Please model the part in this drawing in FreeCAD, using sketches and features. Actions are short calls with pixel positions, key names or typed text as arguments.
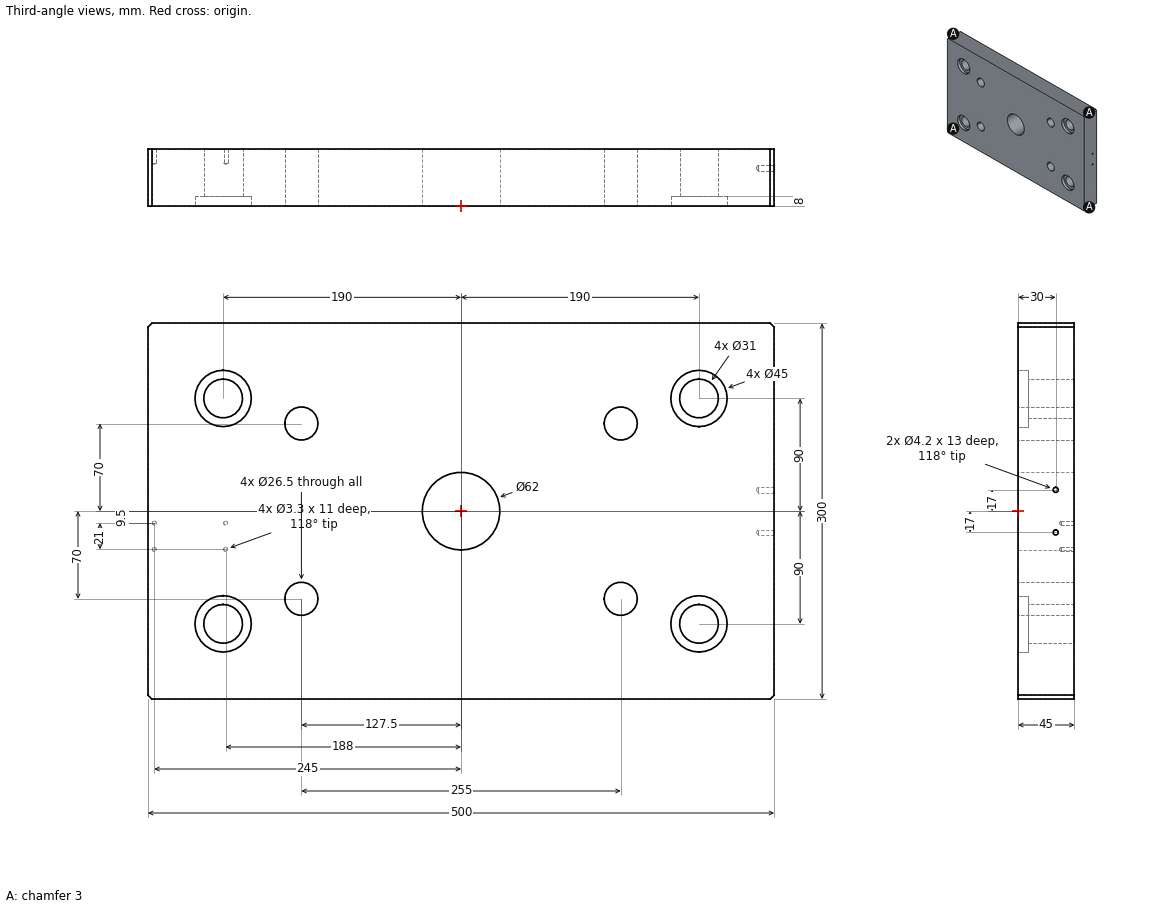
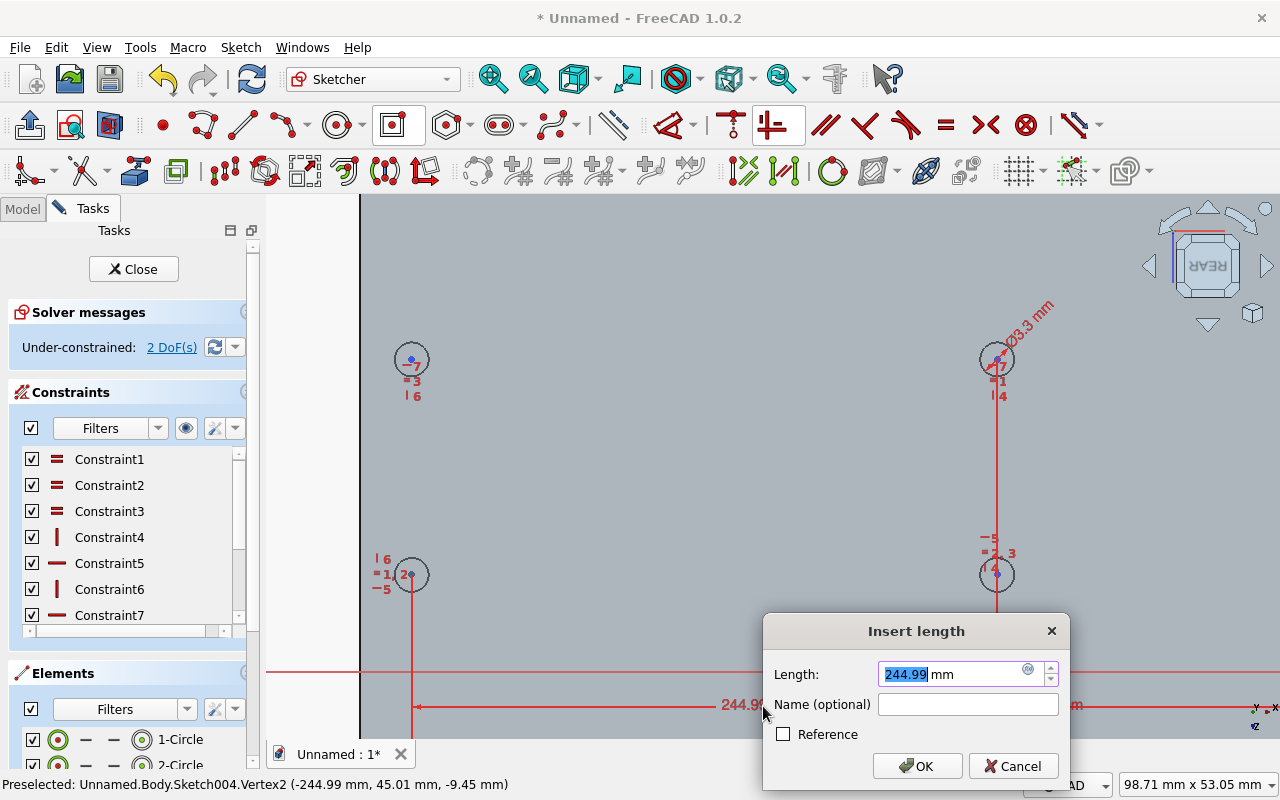
text(245)
key(Return)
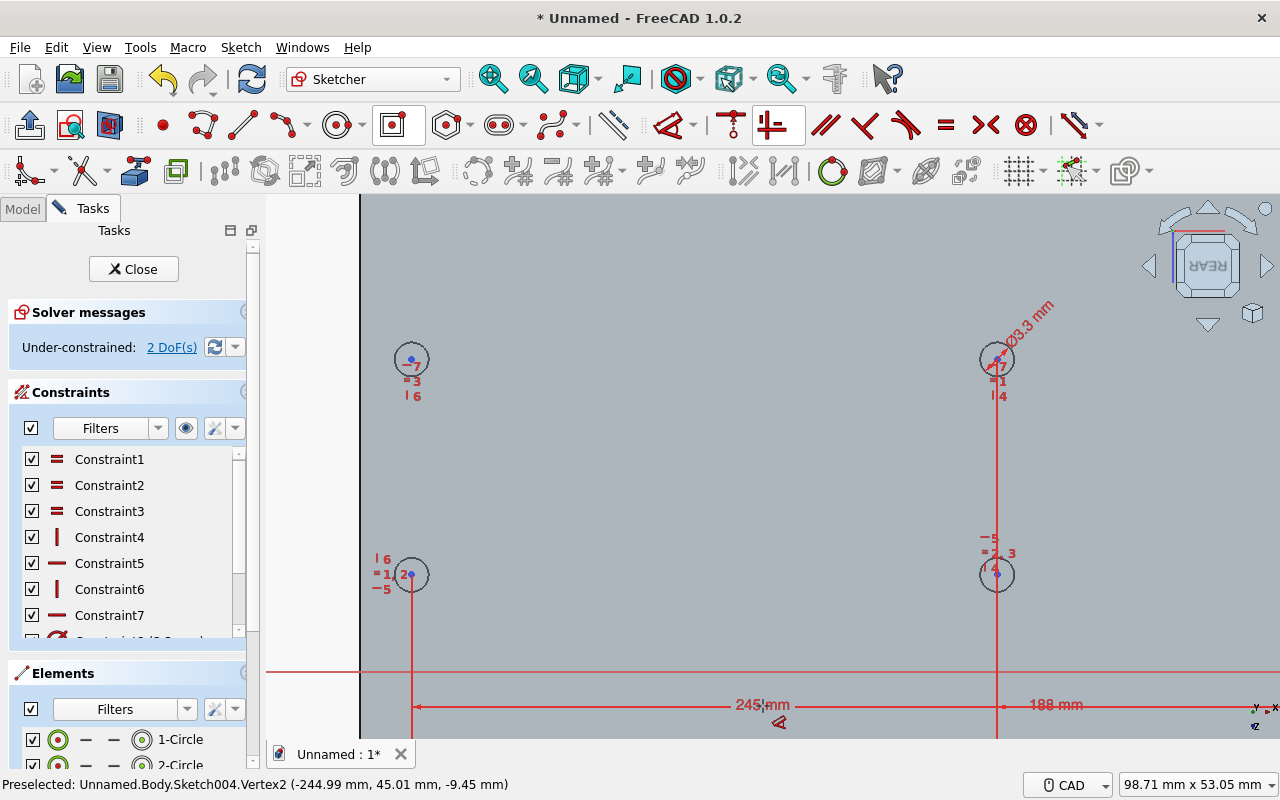
click(412, 575)
click(378, 623)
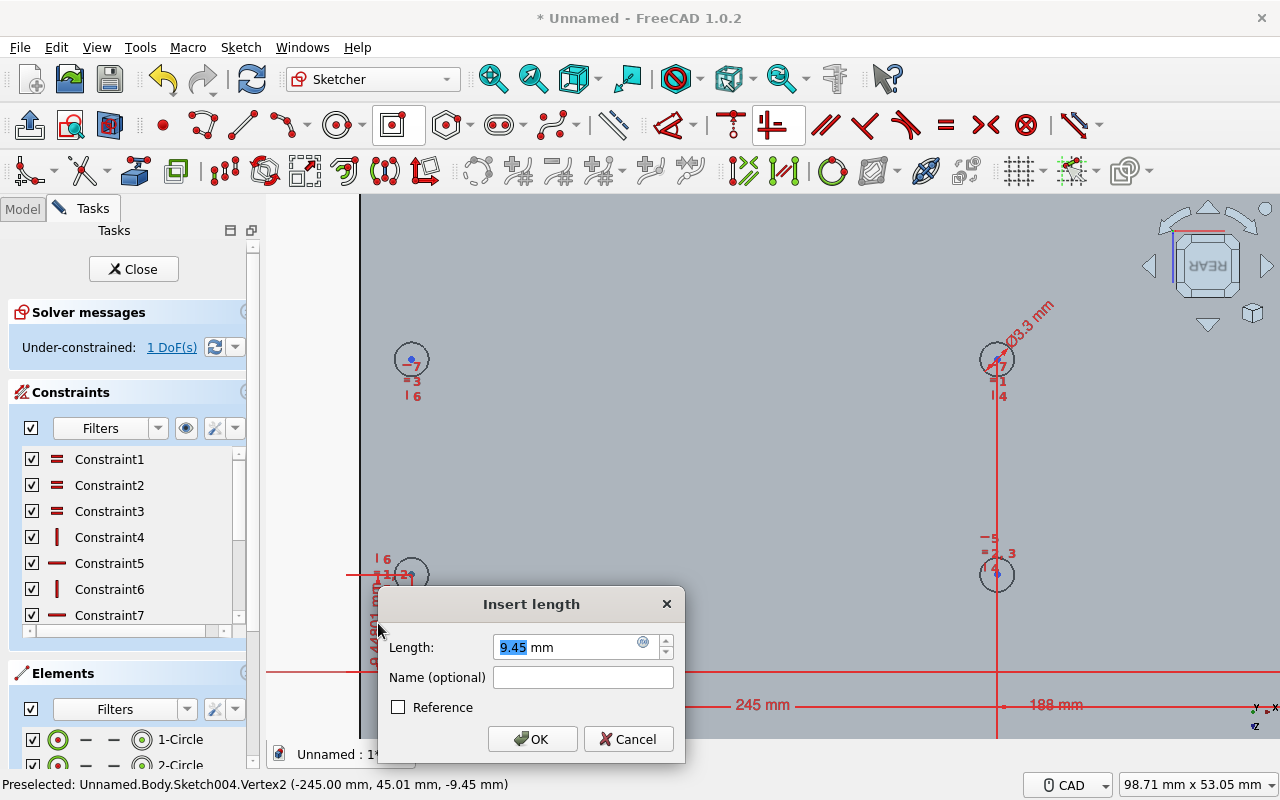
text(9.5)
key(Return)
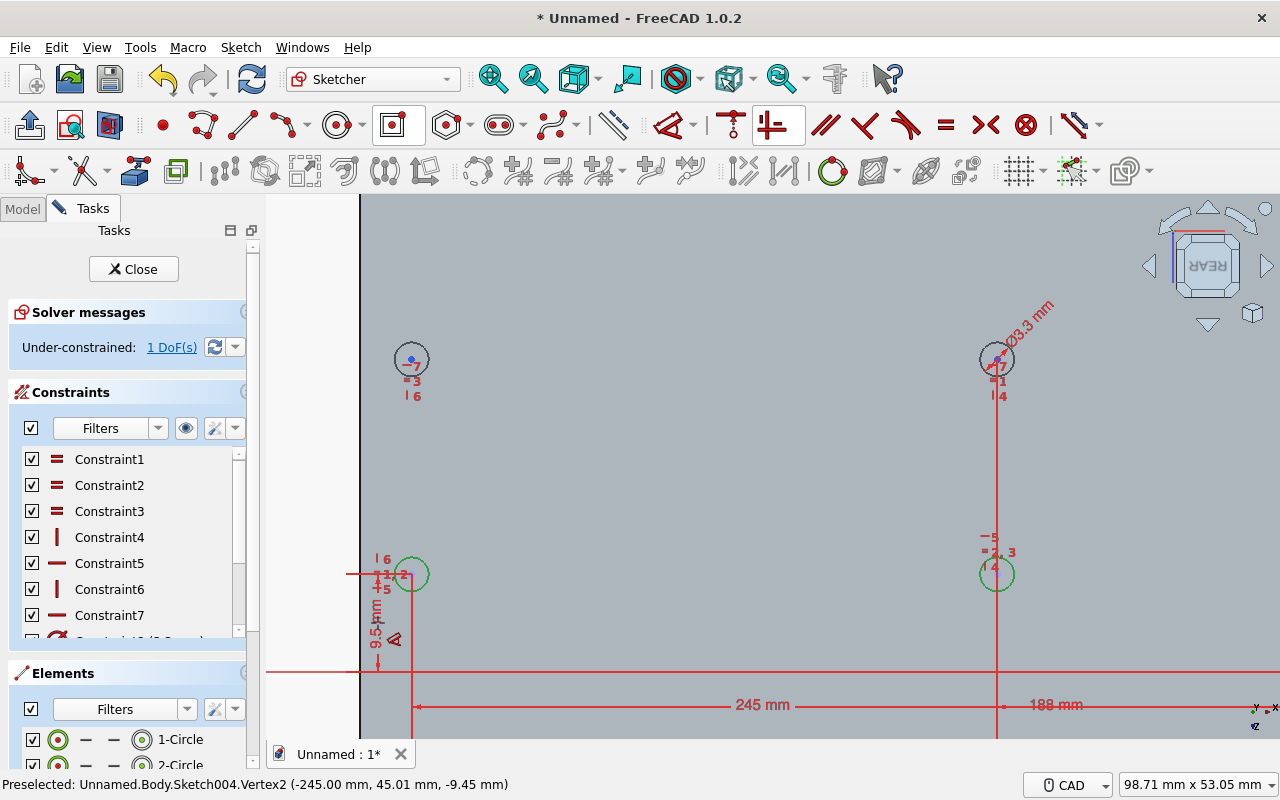
click(997, 359)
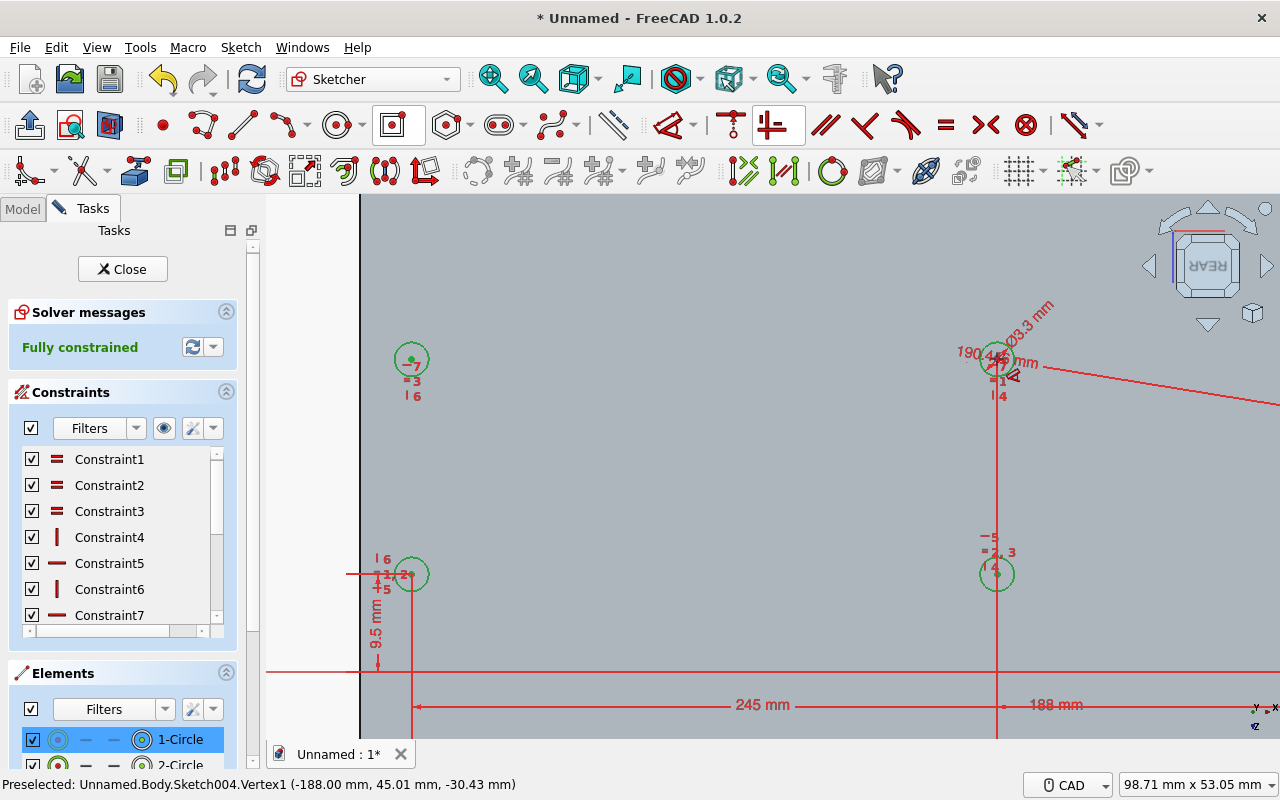
click(412, 574)
click(378, 467)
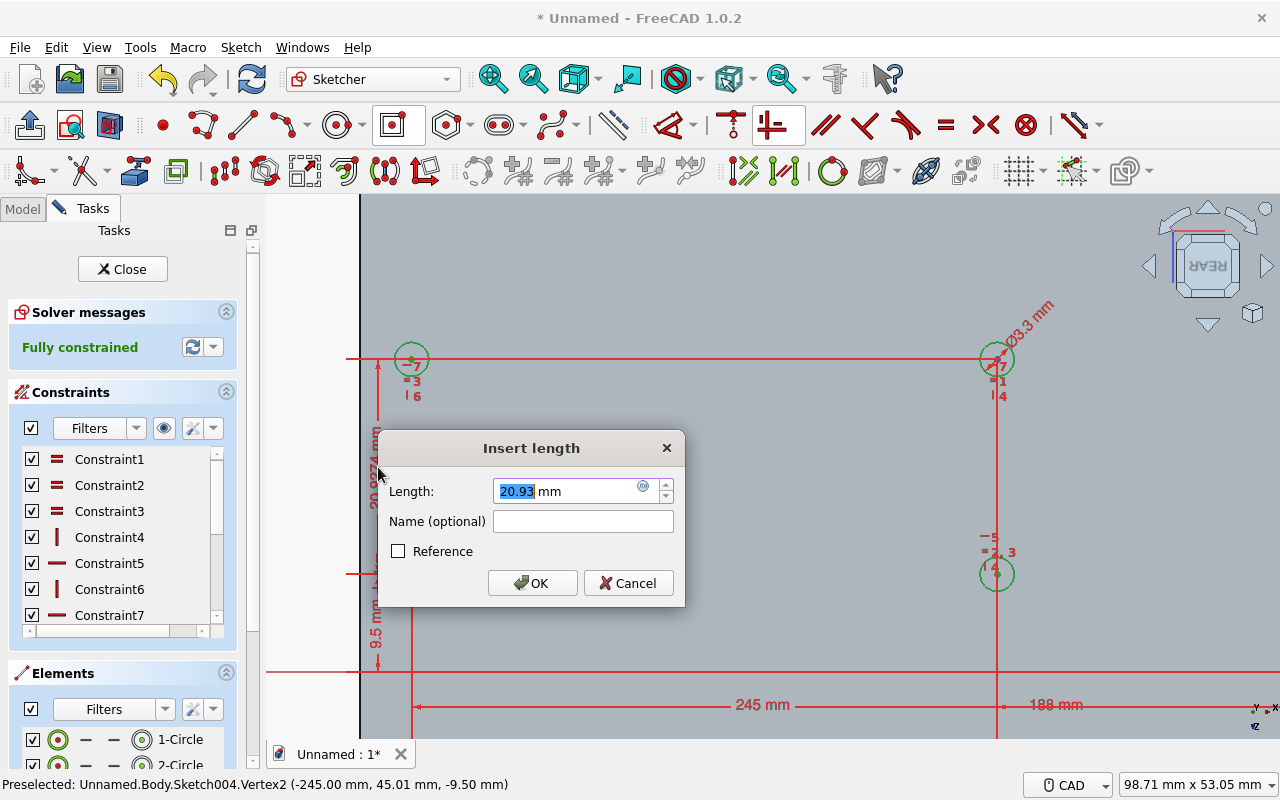
text(21)
key(Return)
key(Escape)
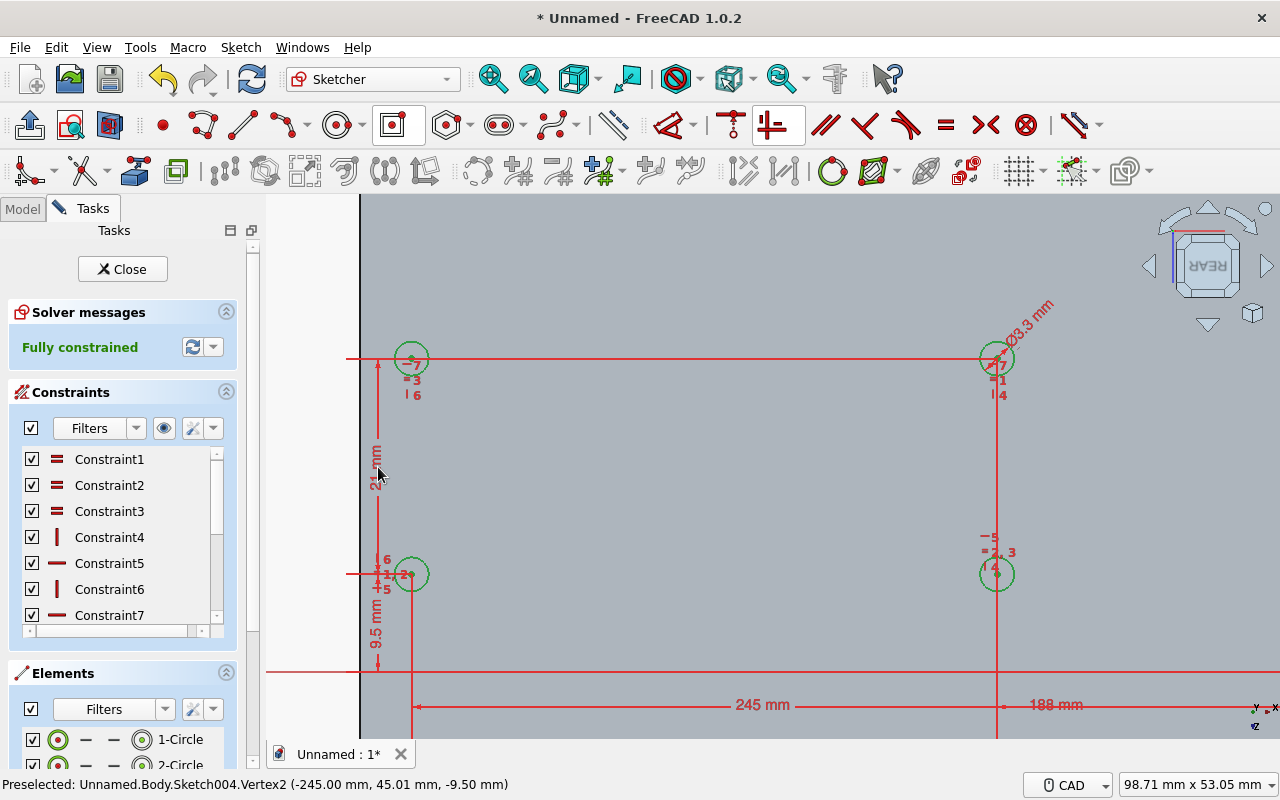
click(123, 269)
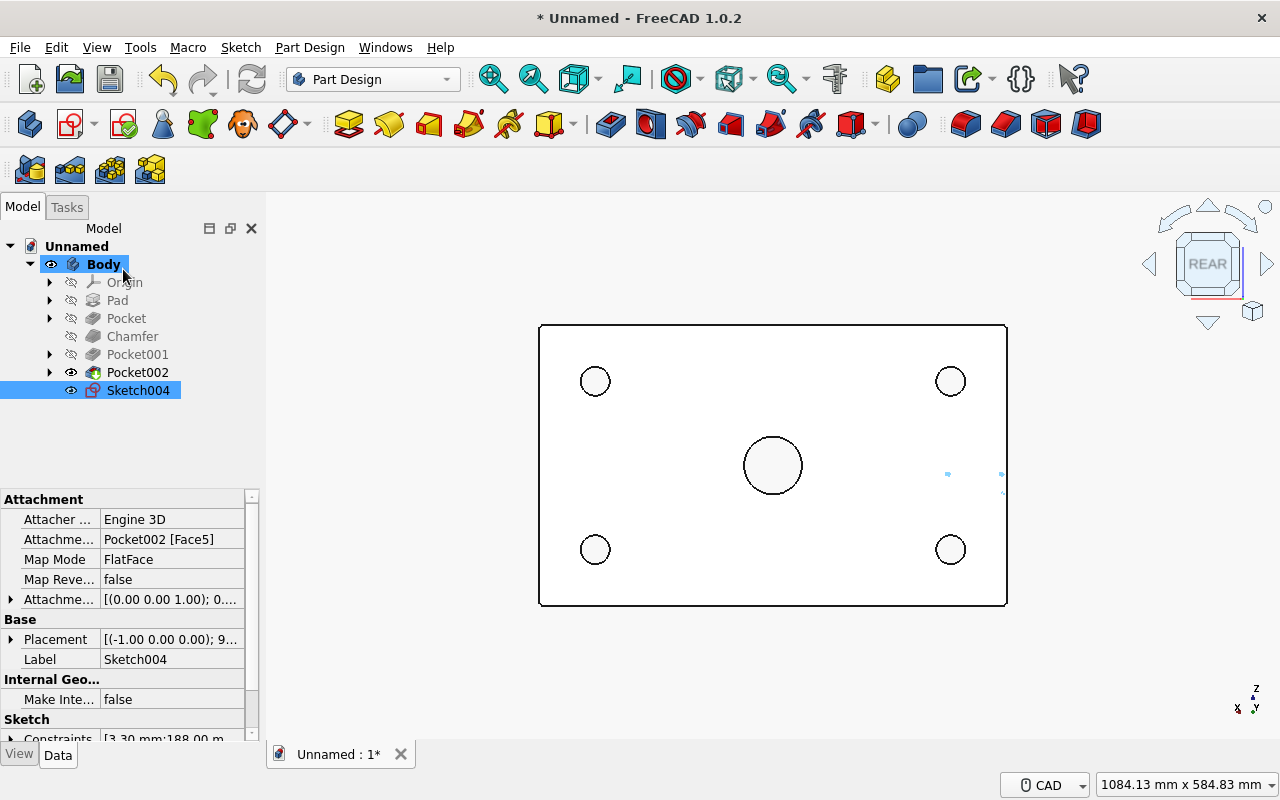
click(652, 124)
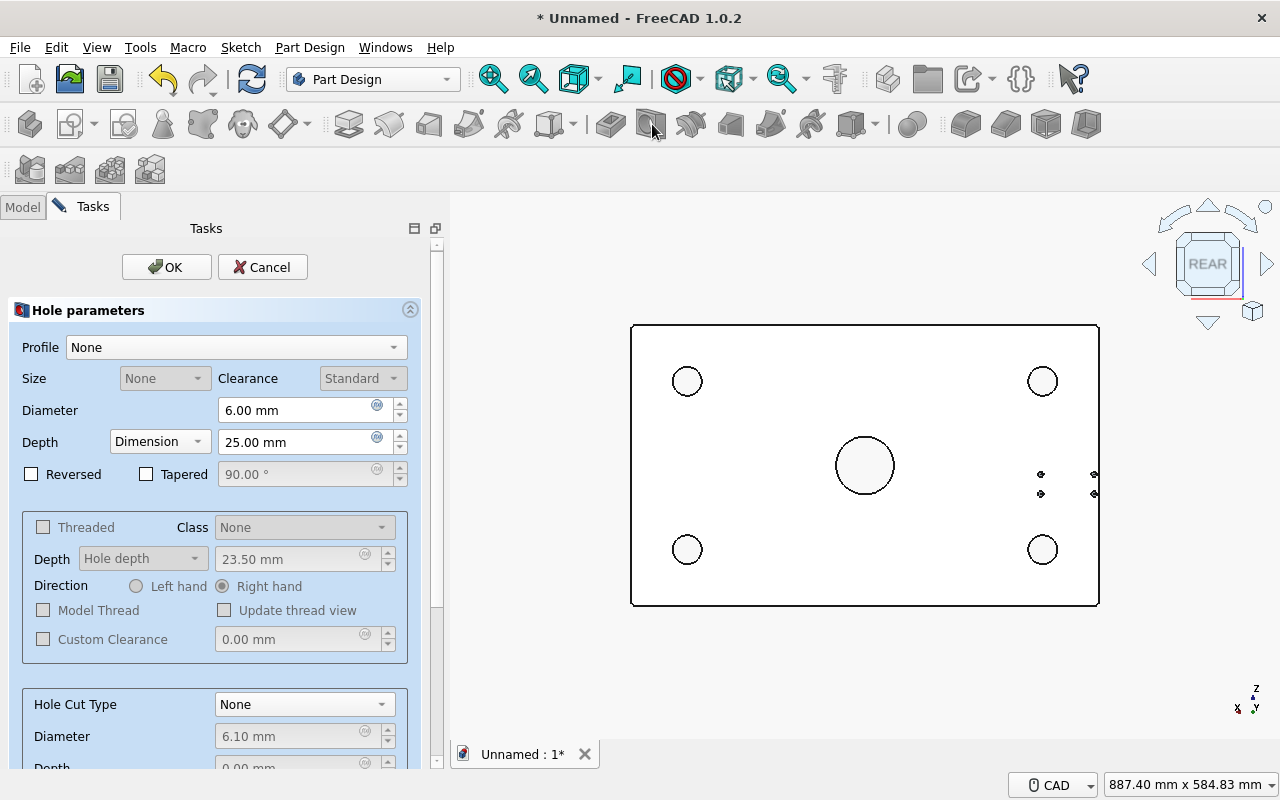
triple_click(305, 410)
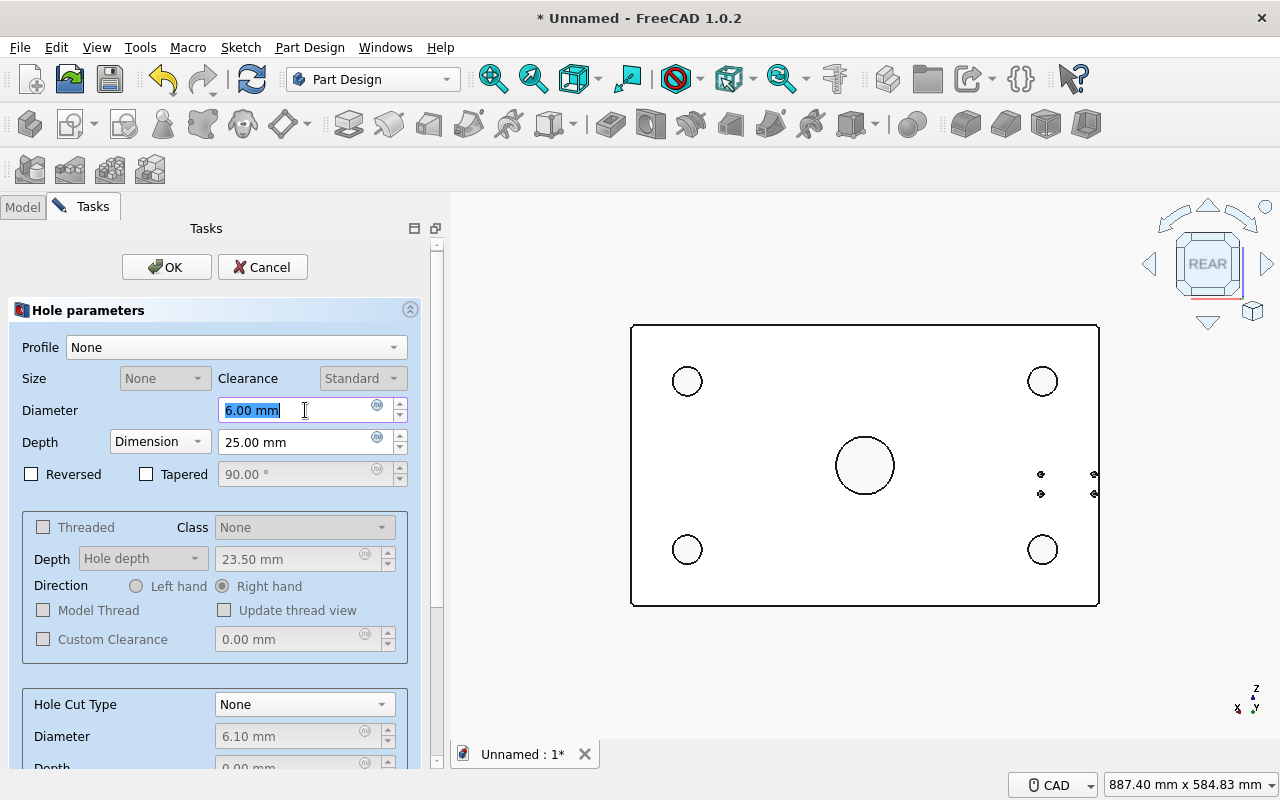
text(3.3)
key(Tab)